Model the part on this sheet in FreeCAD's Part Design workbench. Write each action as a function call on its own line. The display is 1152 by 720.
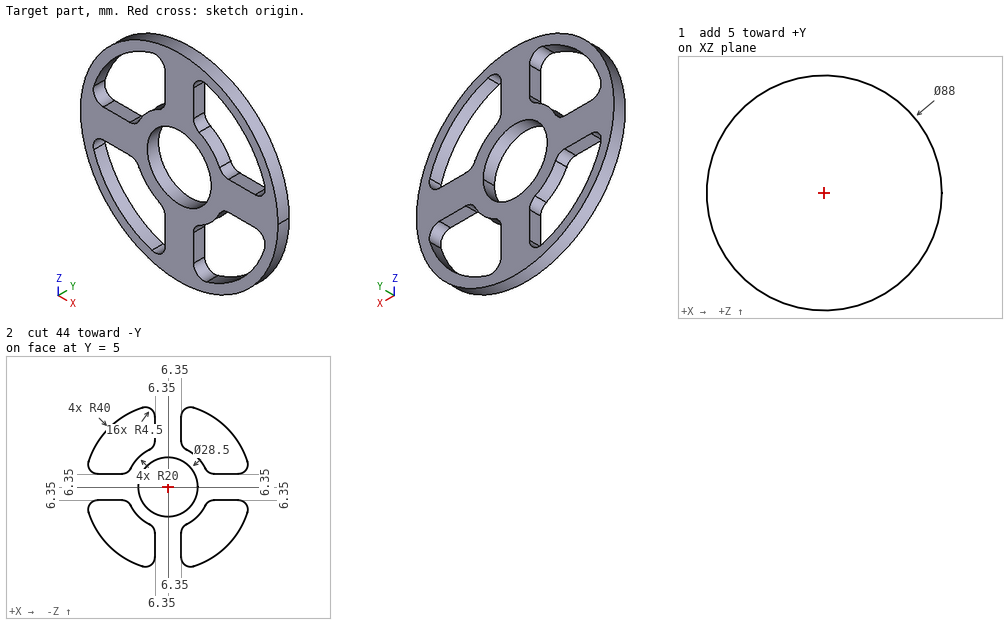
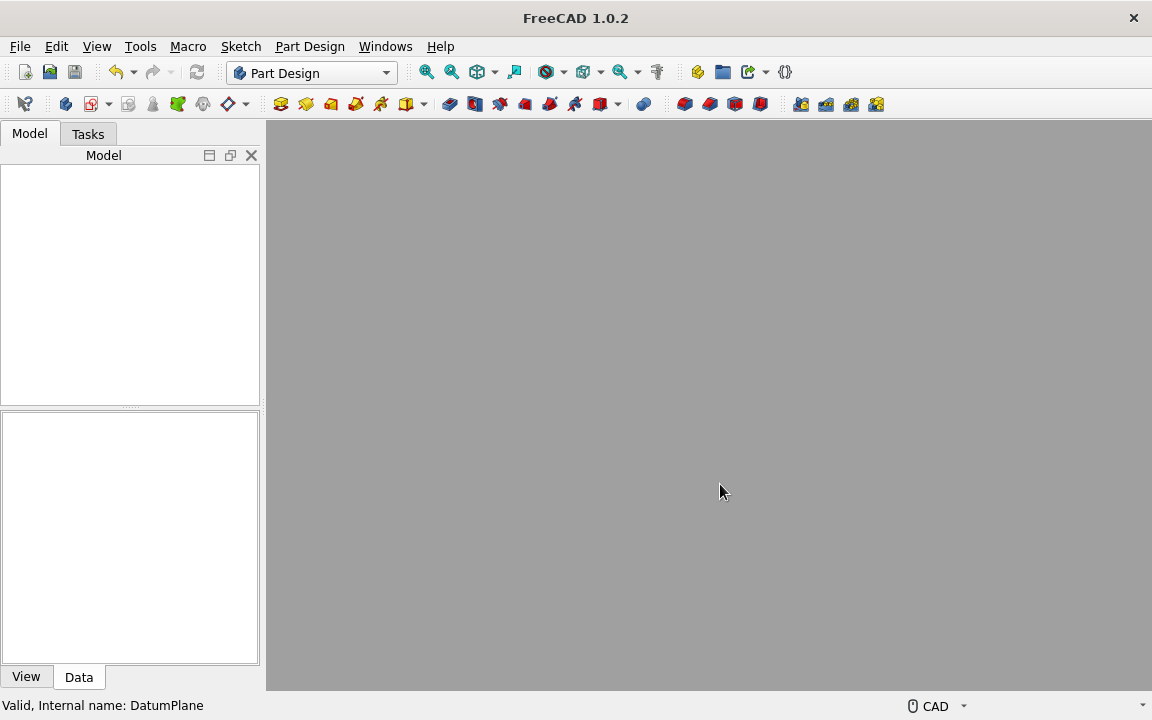
key(ctrl+n)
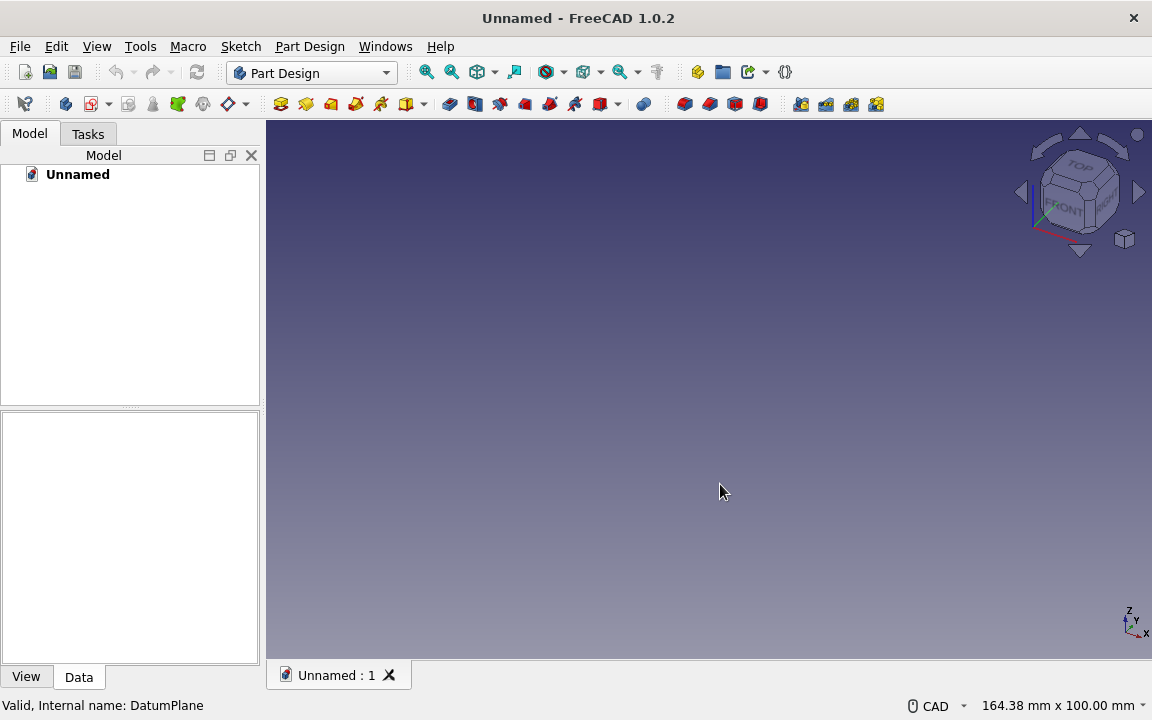
click(90, 104)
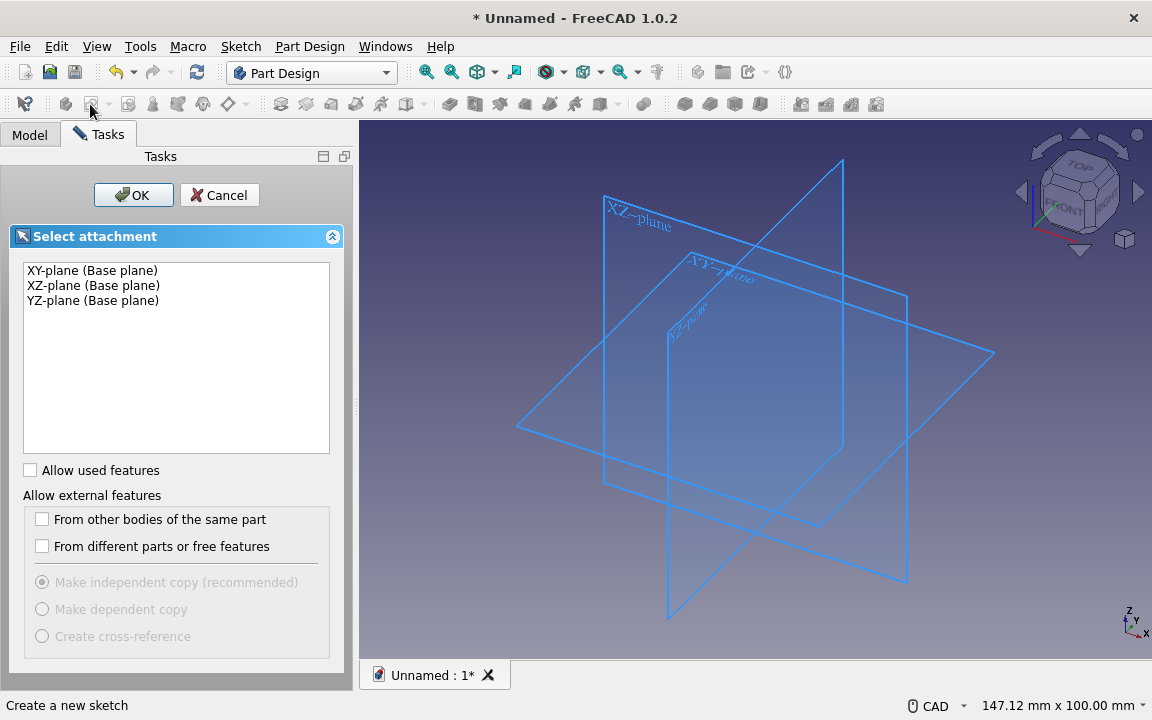
click(84, 286)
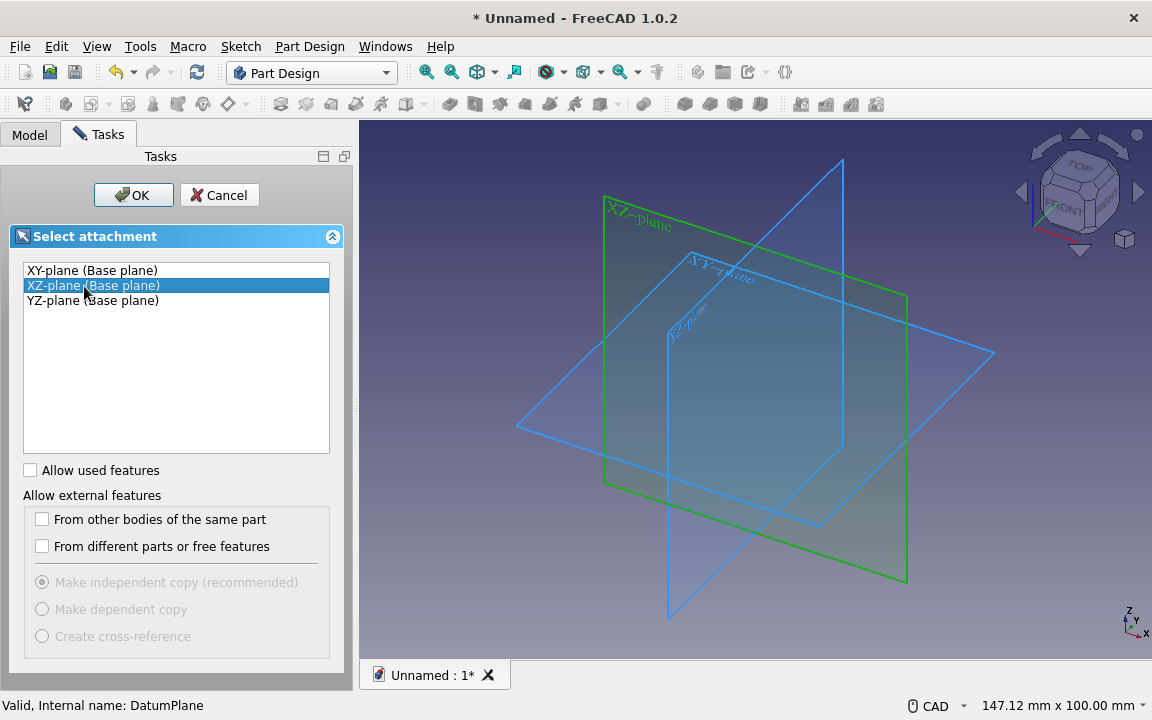
click(134, 195)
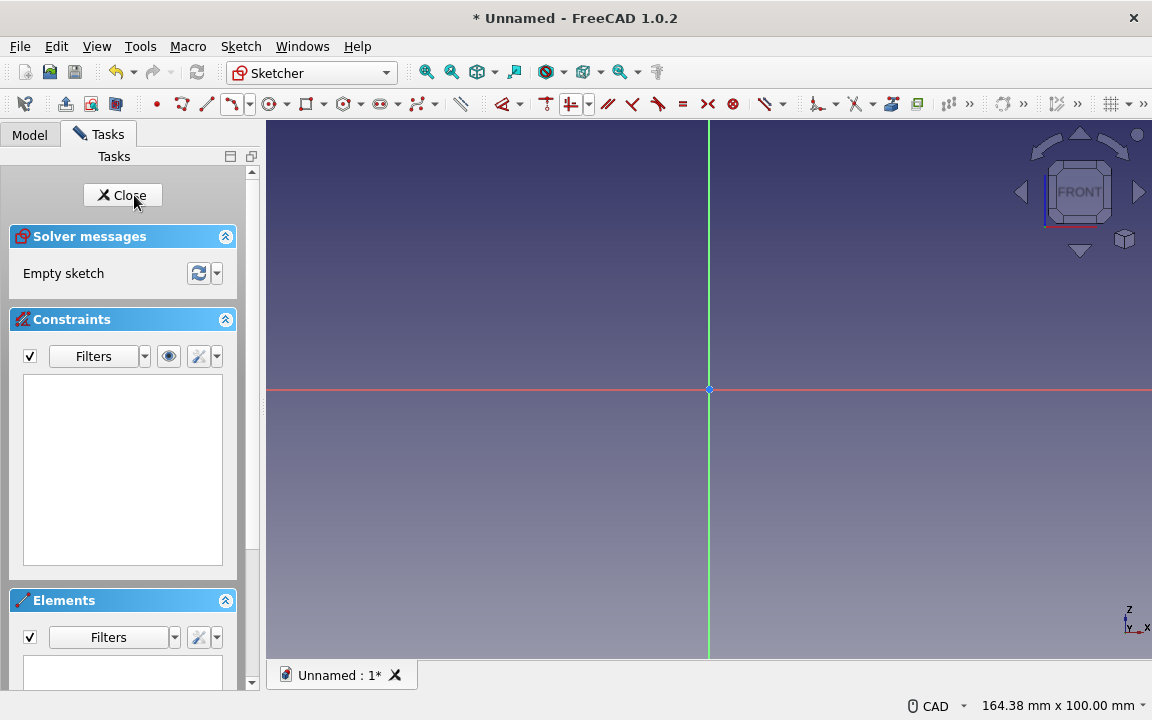
scroll(501, 390, down, 2)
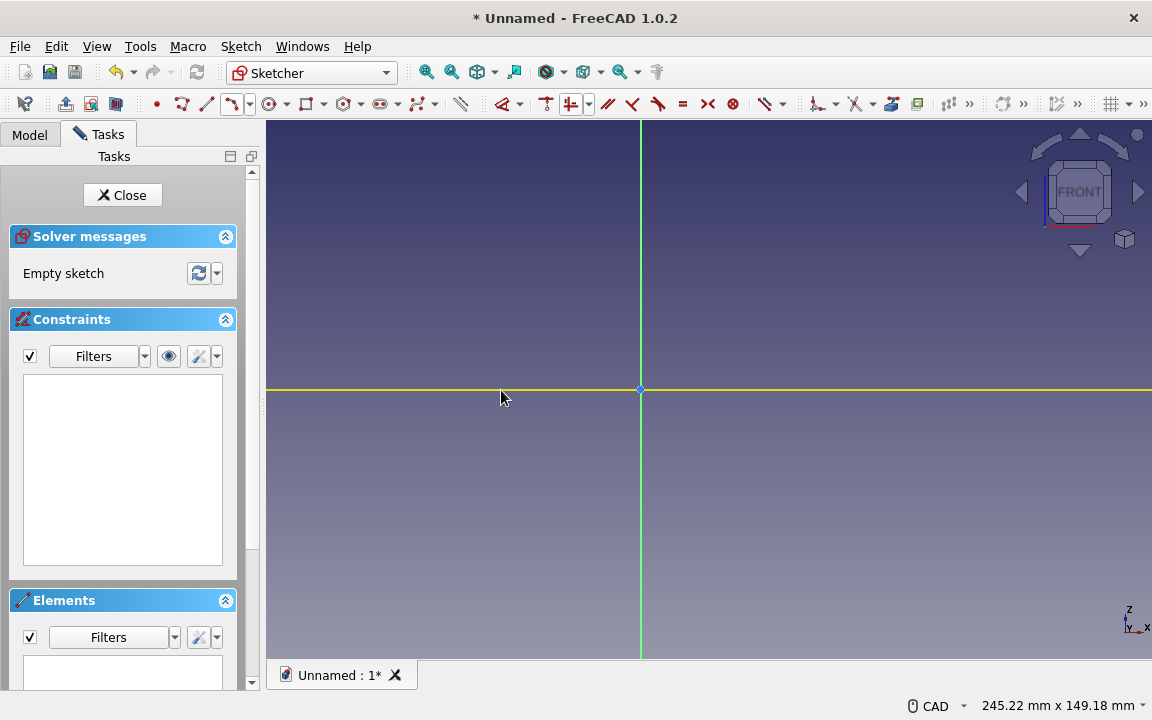
key(g)
key(c)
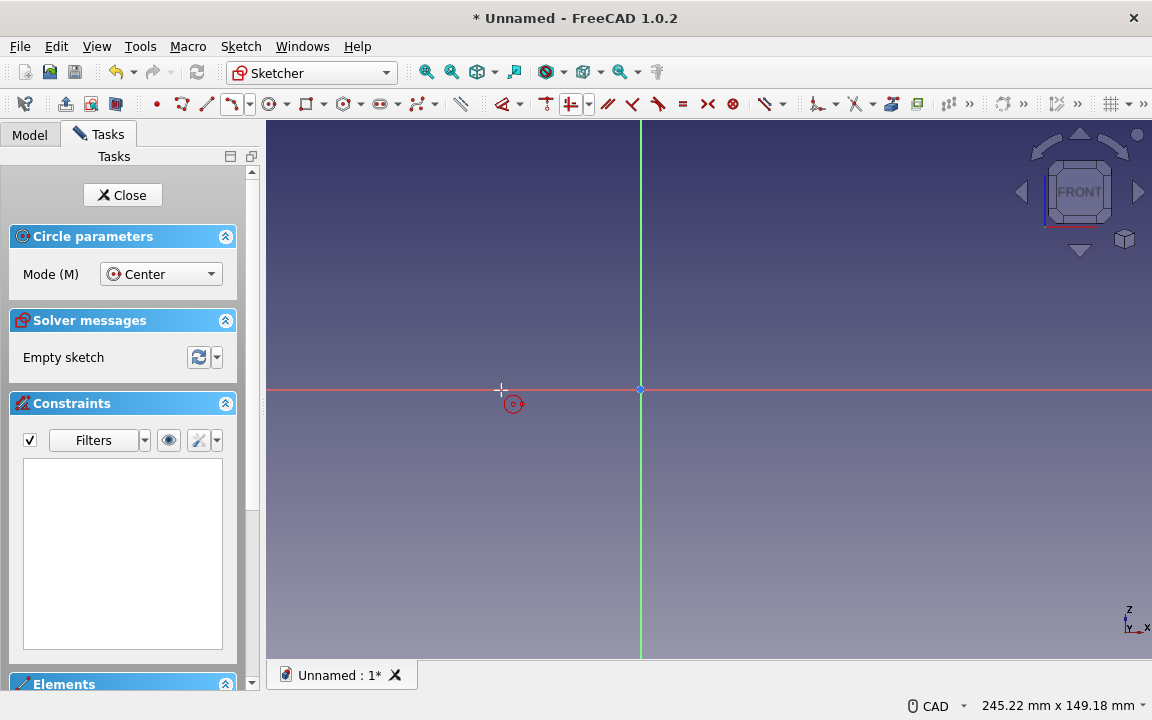
click(641, 390)
move(753, 277)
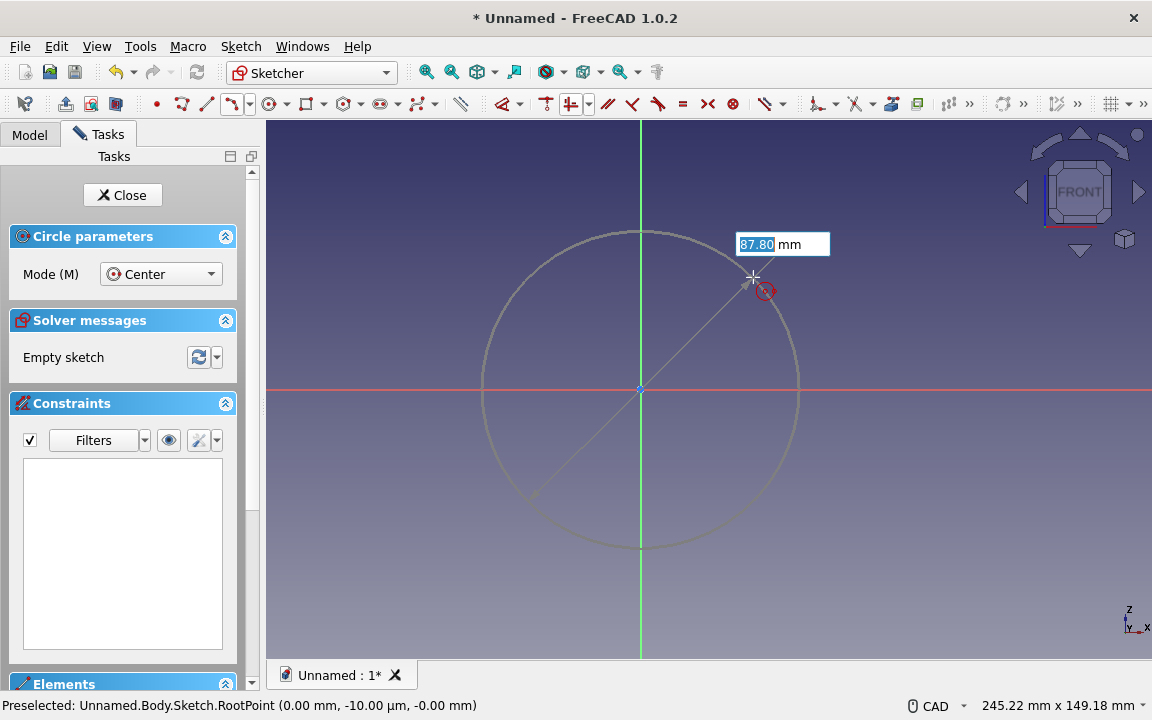
text(88)
key(Return)
key(Escape)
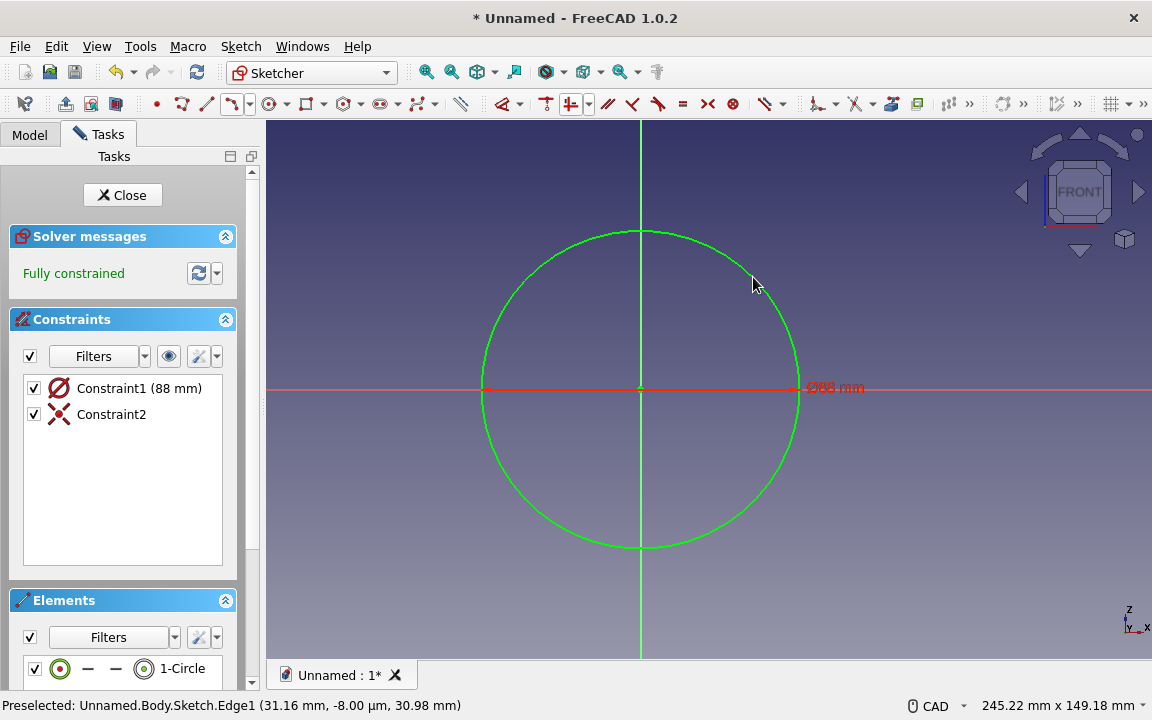
click(123, 195)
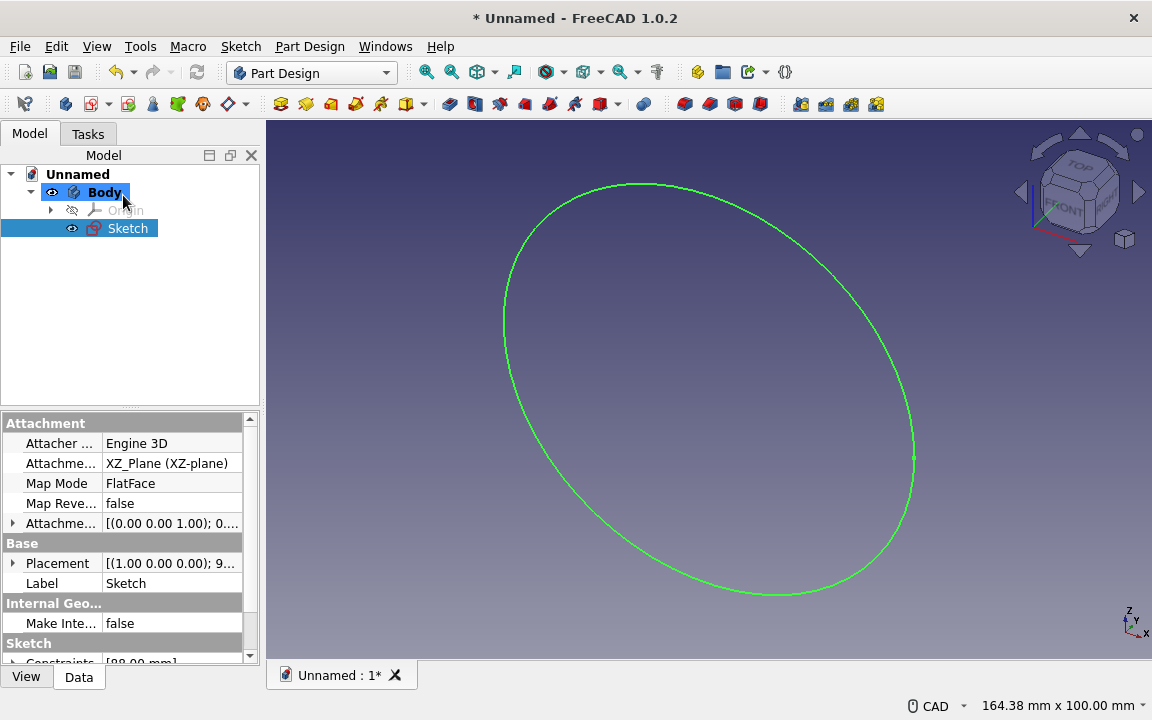
click(281, 104)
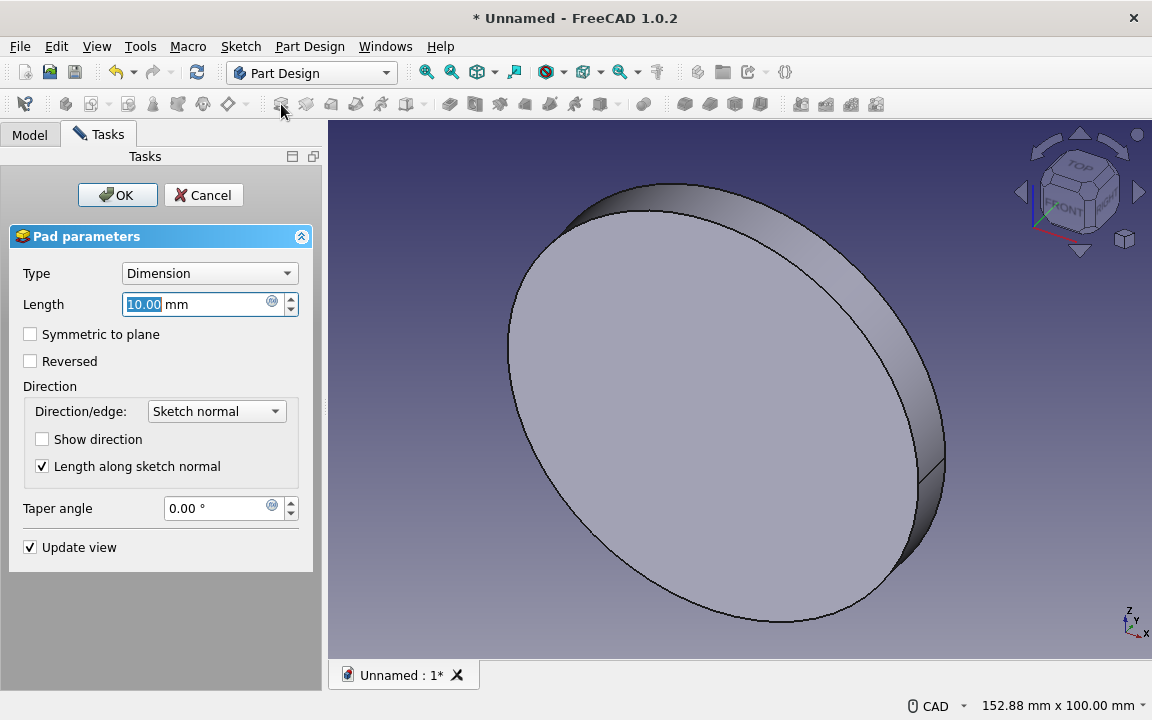
text(5)
key(Tab)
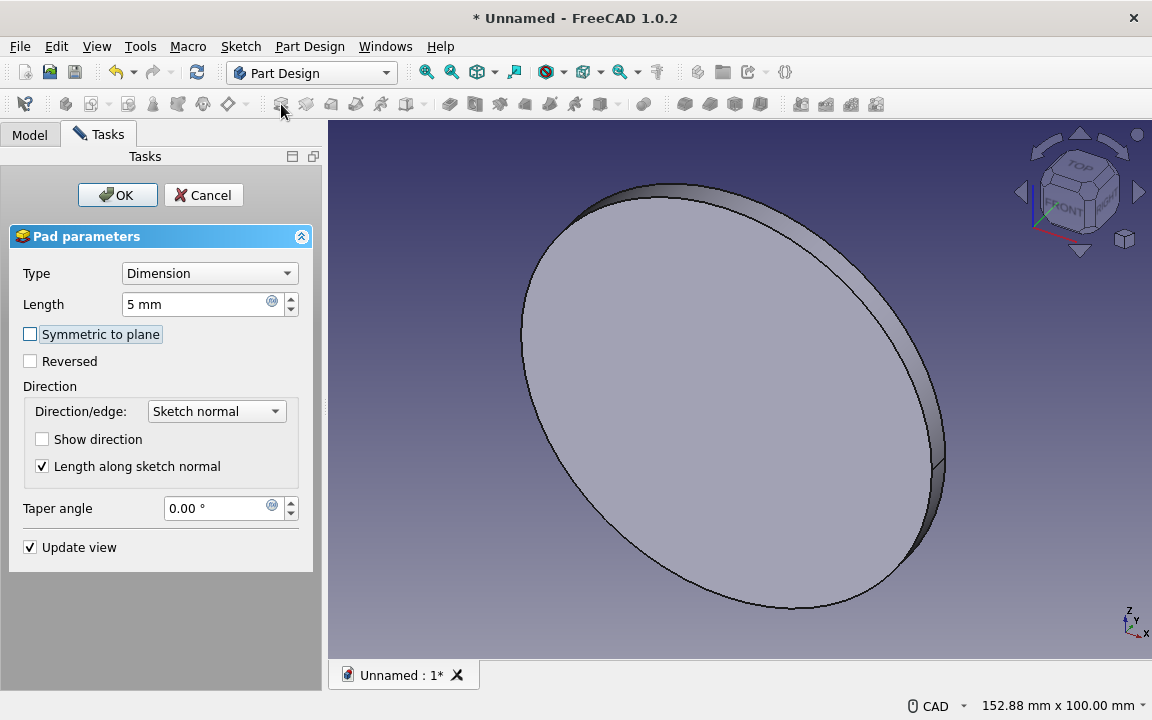
click(31, 361)